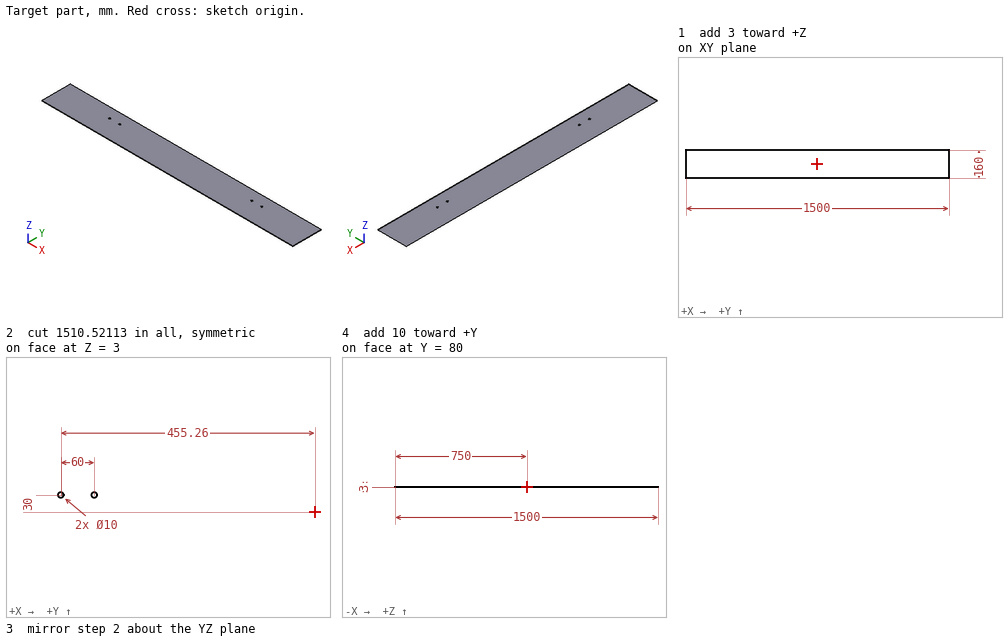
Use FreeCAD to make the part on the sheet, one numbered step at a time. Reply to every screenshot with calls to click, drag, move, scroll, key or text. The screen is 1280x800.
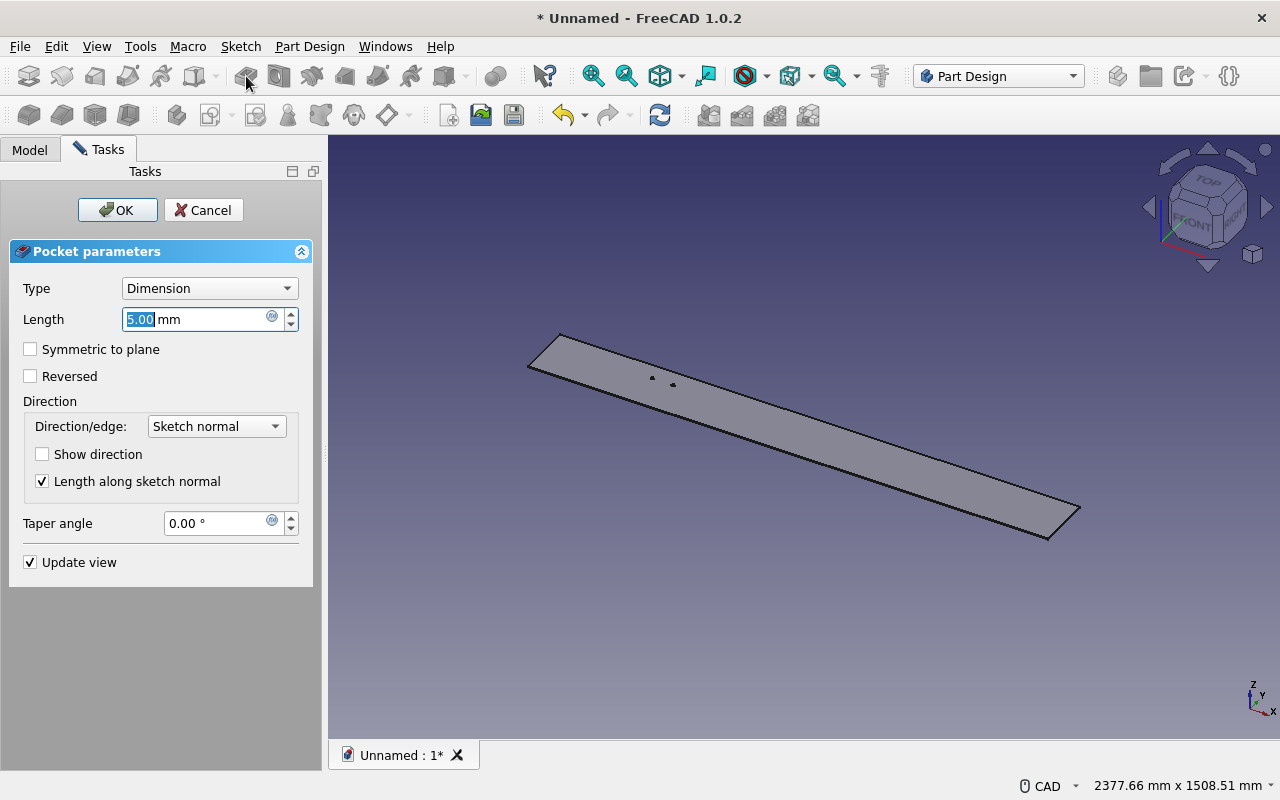
text(1510.52113)
key(Tab)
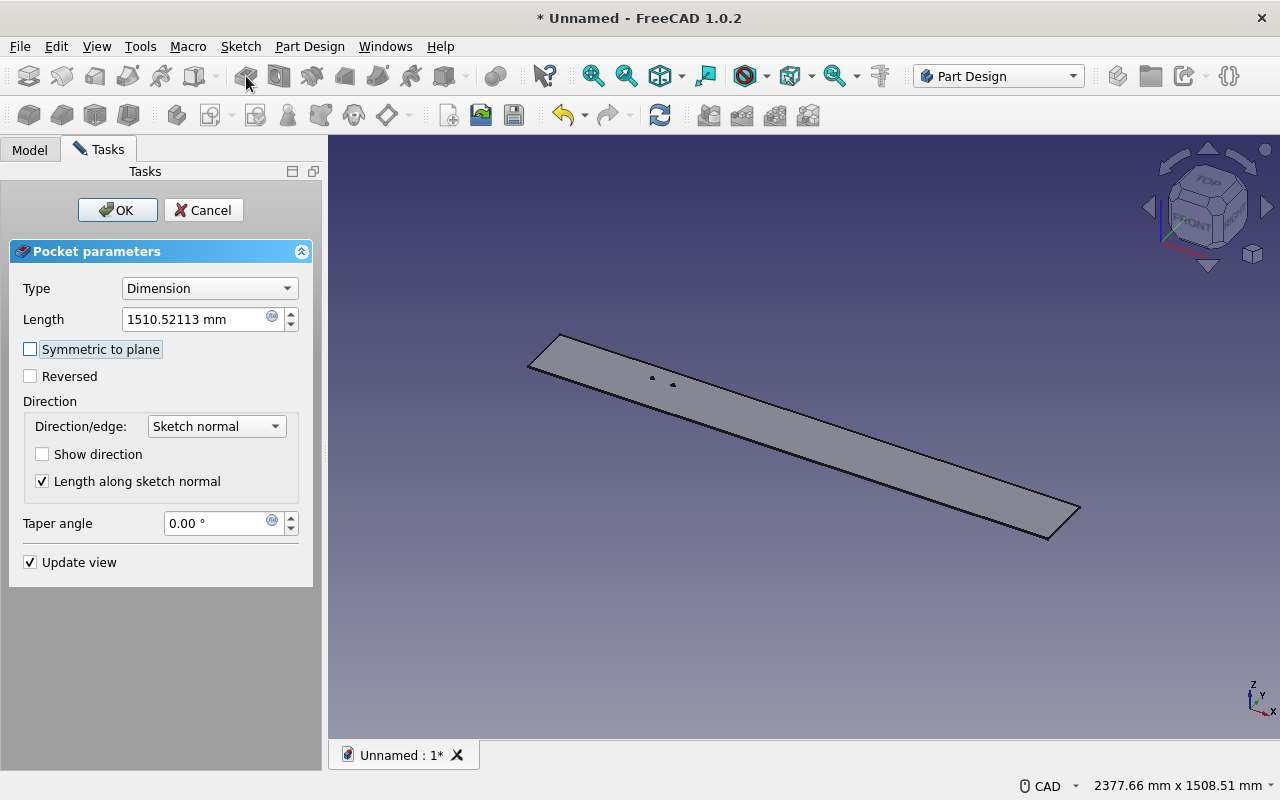
click(31, 349)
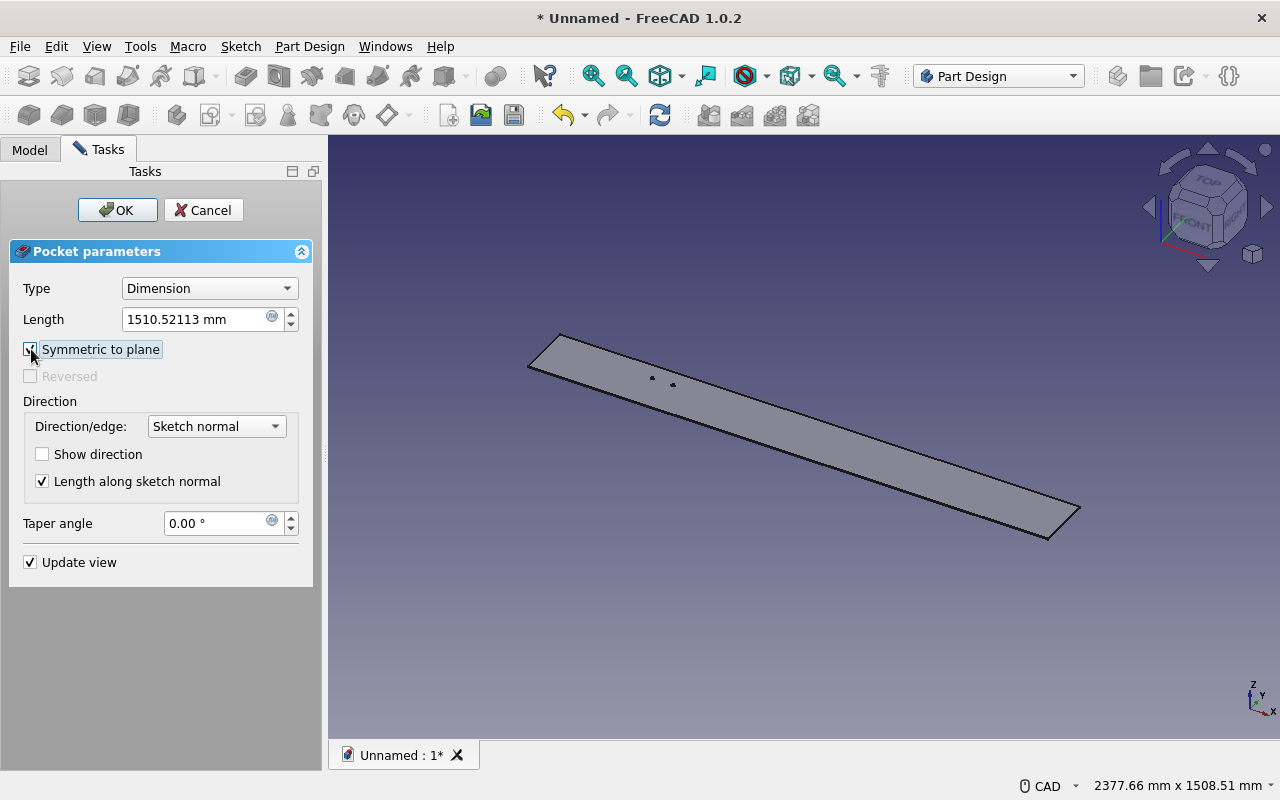
click(118, 210)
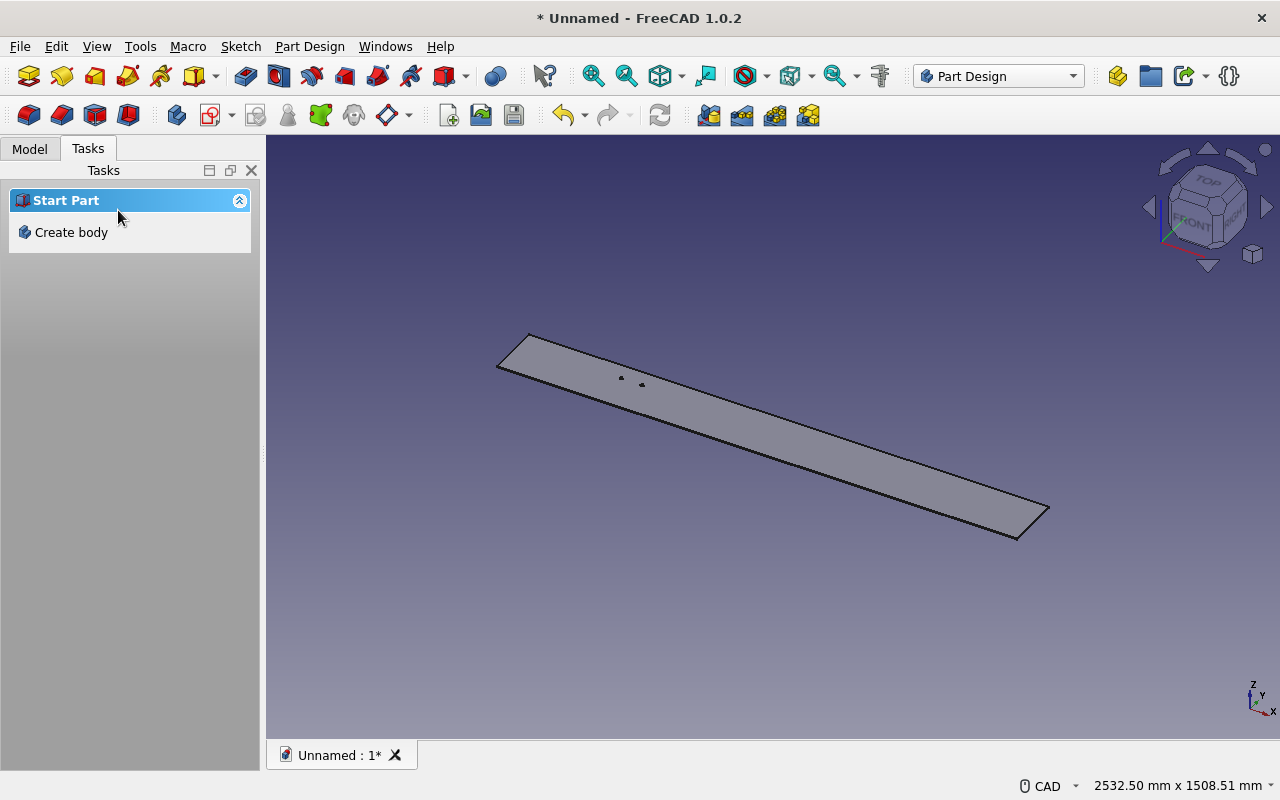
click(30, 148)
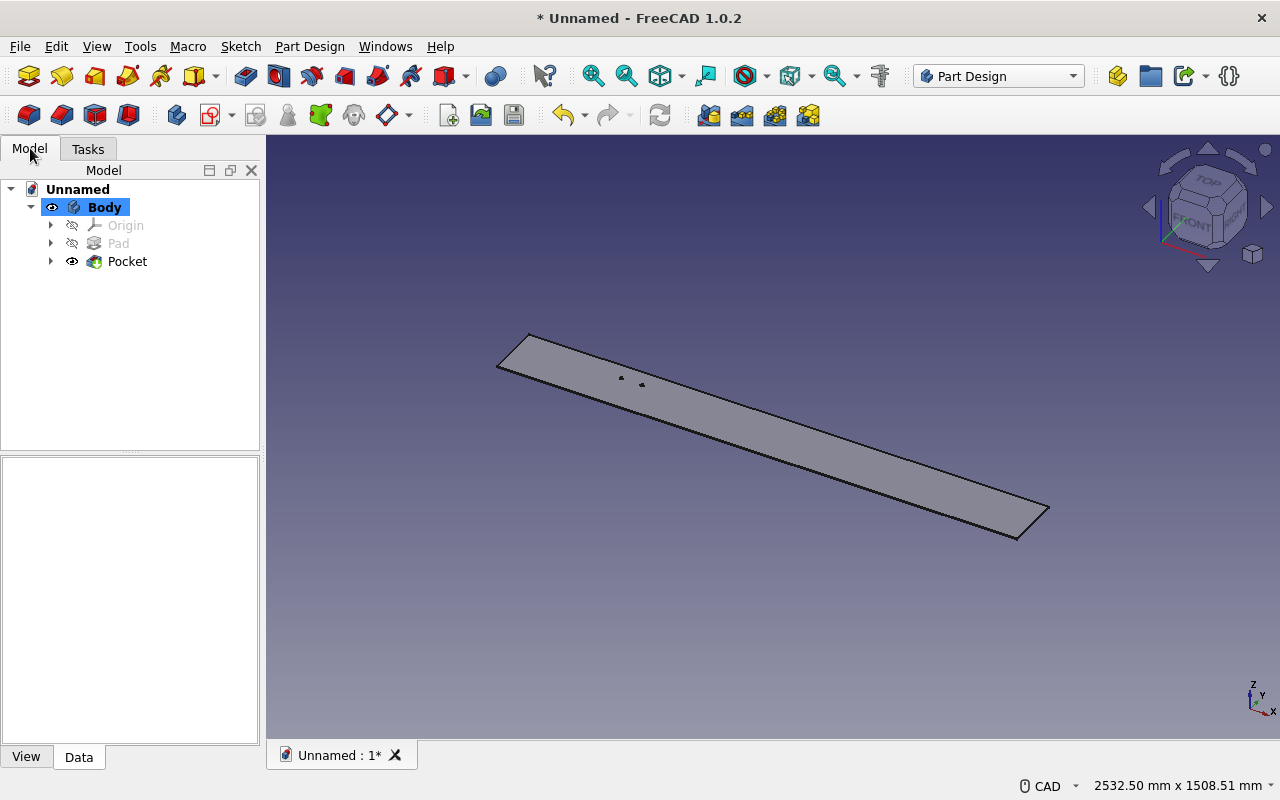
click(117, 261)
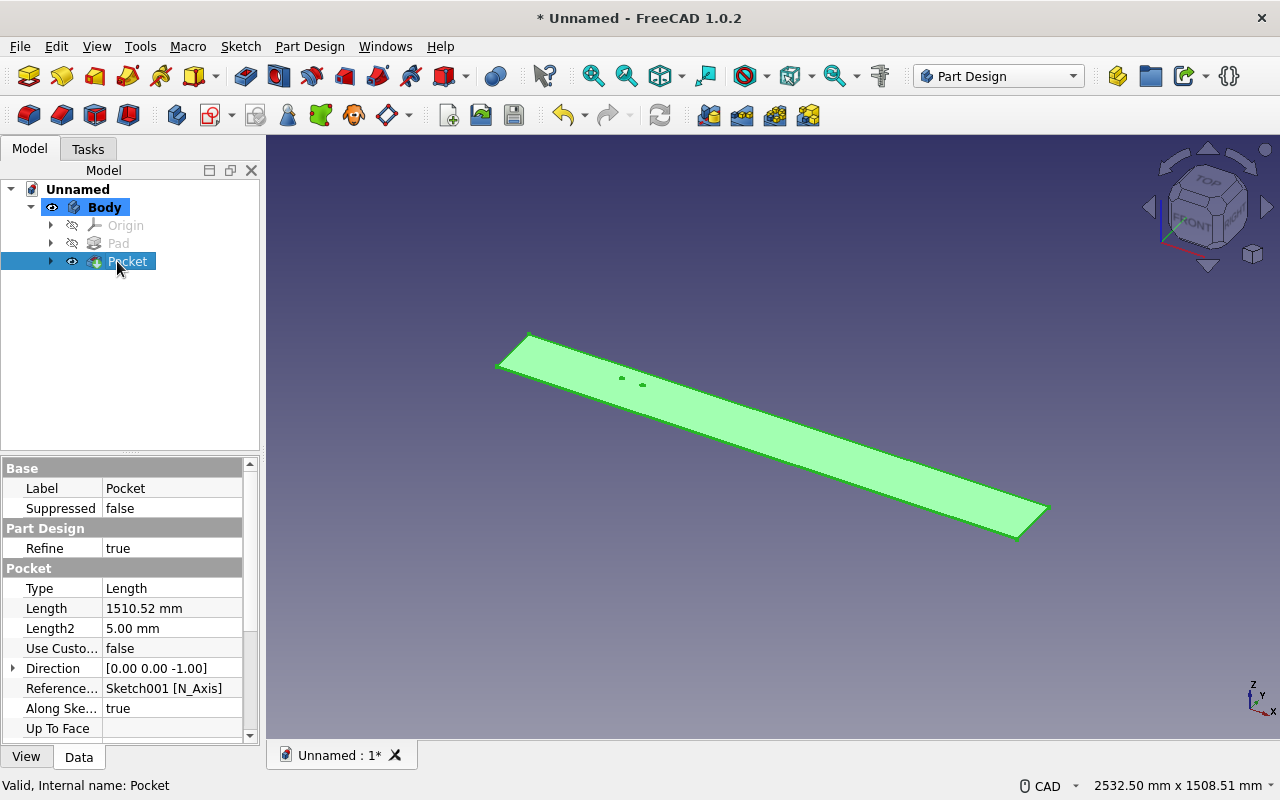
click(709, 116)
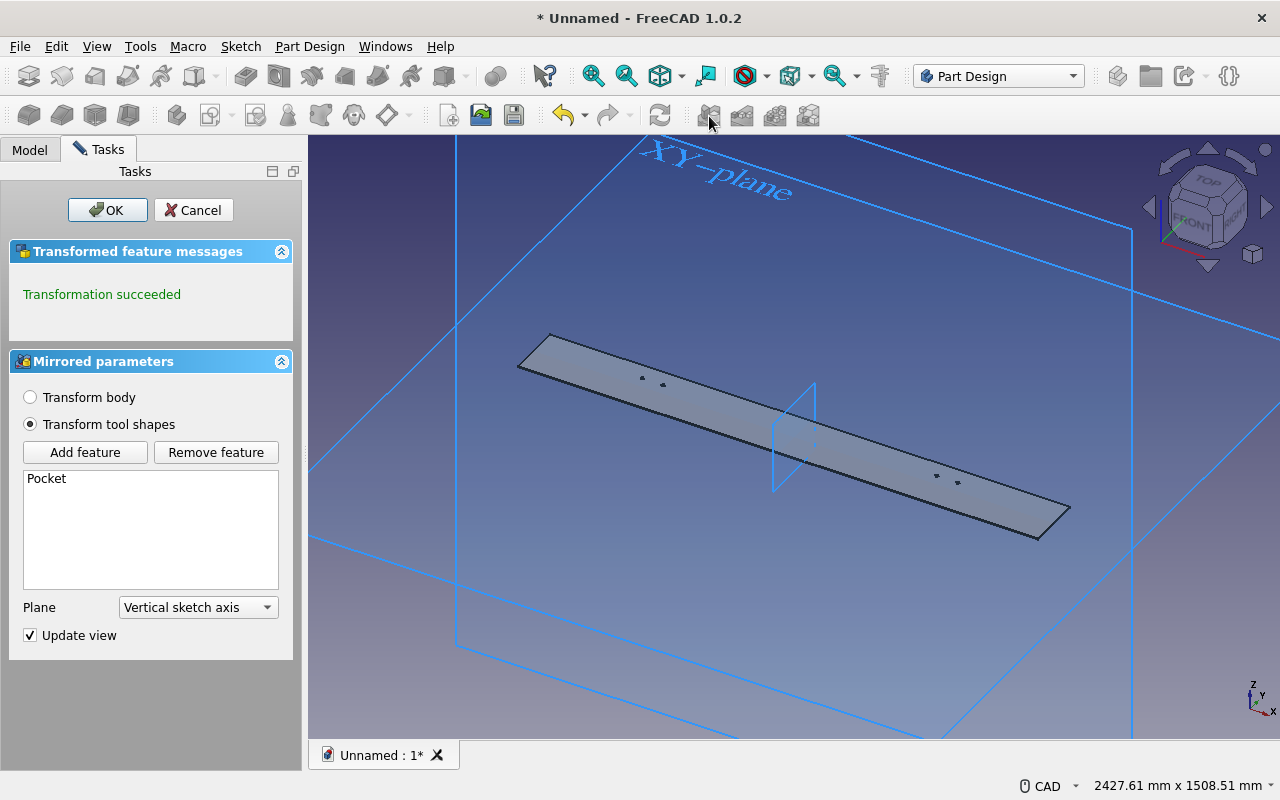
click(199, 608)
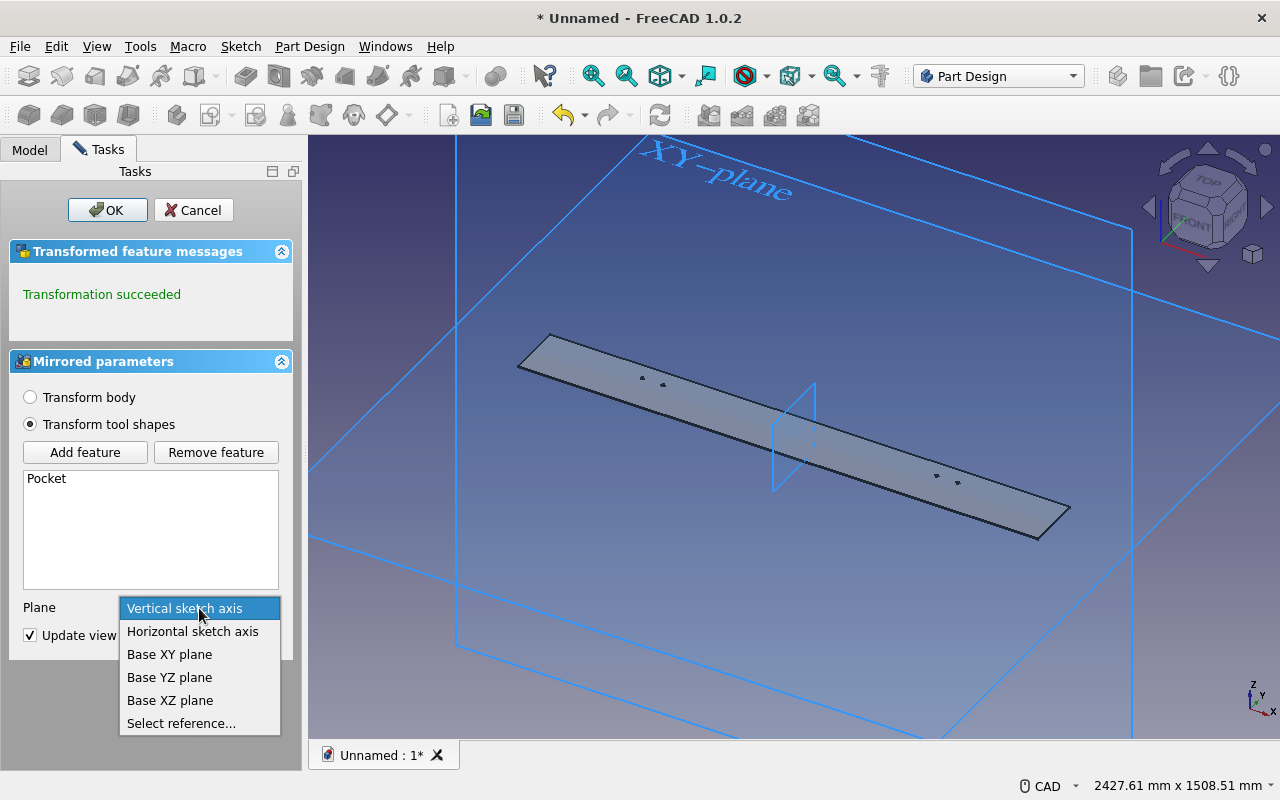
click(198, 678)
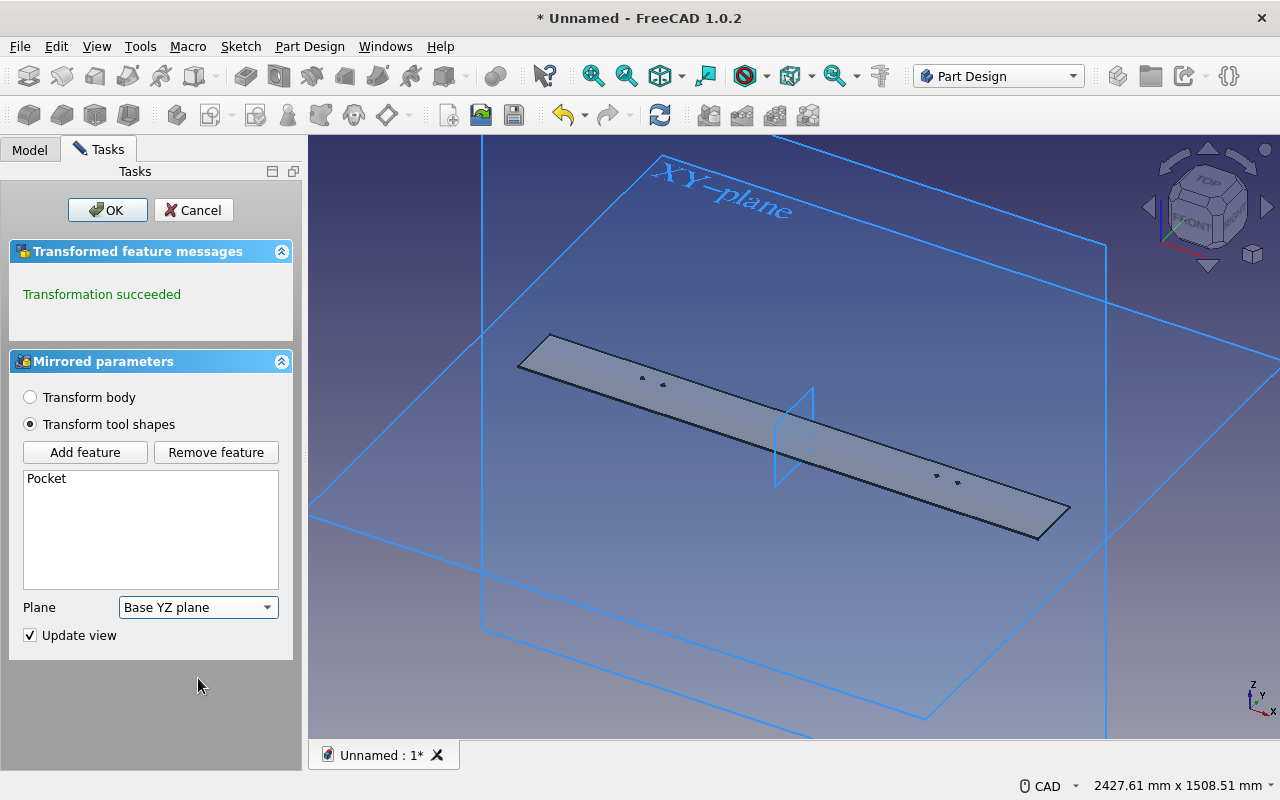
click(108, 210)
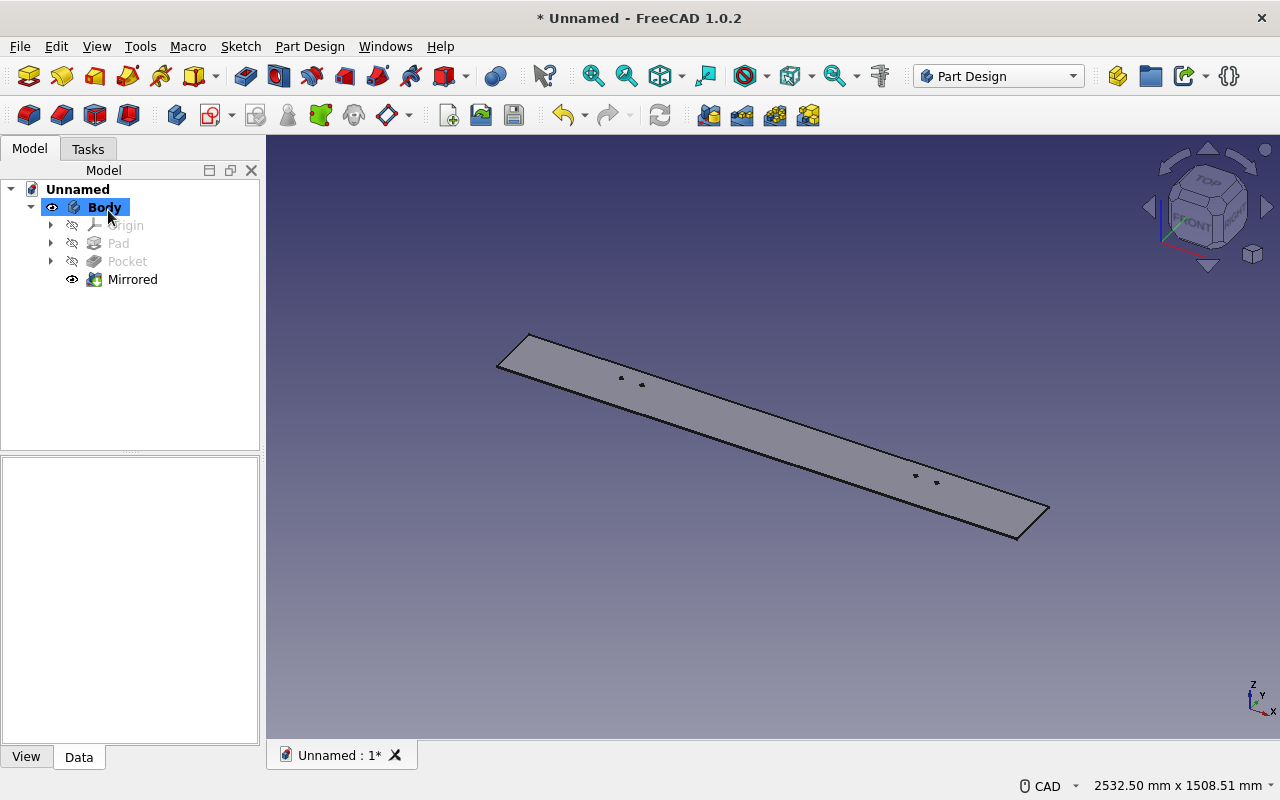
key(4)